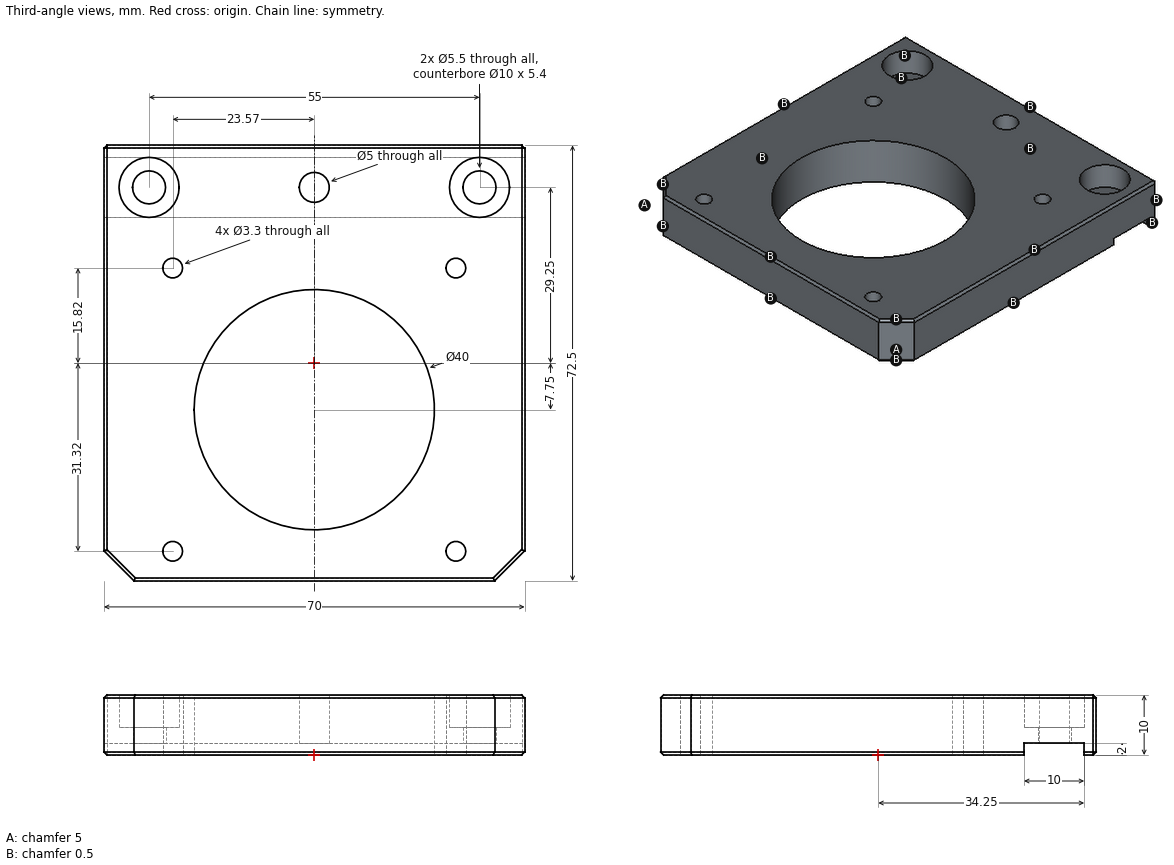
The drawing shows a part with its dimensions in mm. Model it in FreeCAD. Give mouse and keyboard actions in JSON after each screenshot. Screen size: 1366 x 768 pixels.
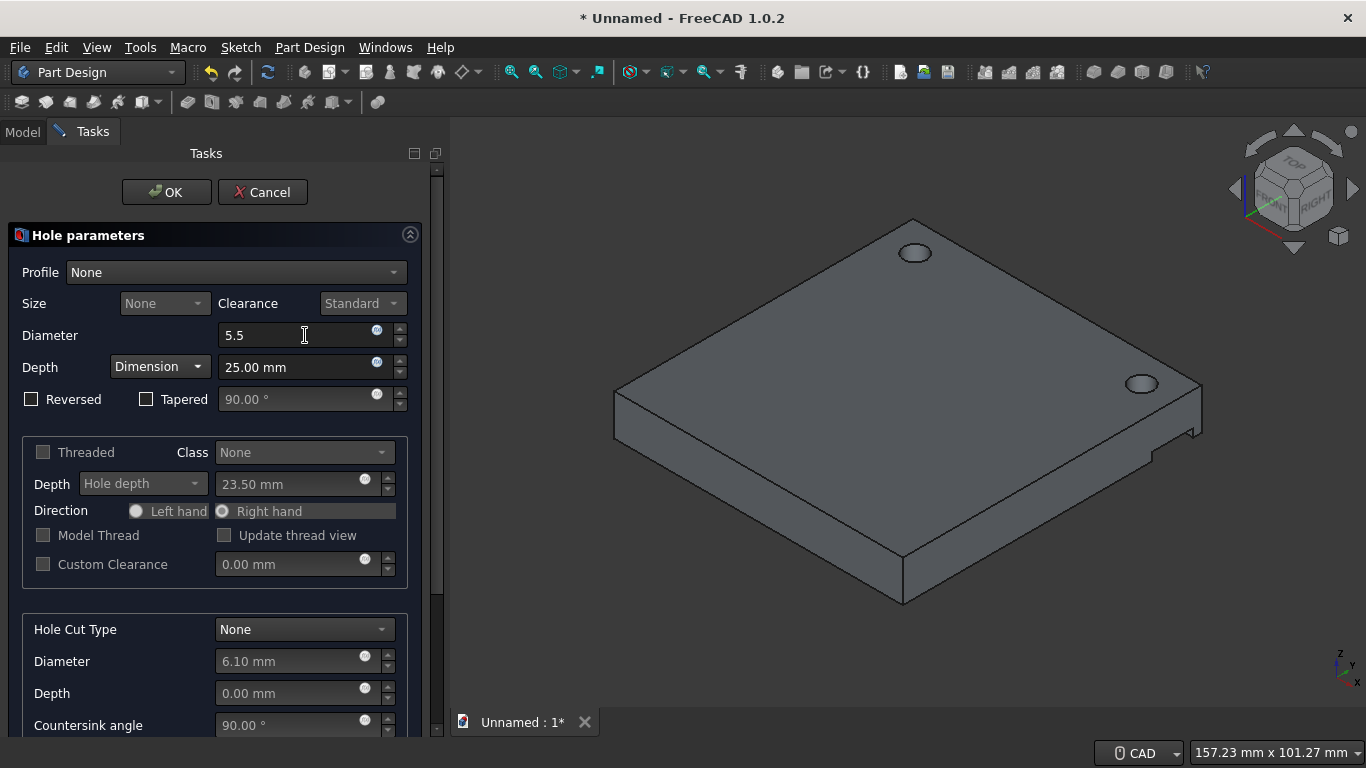
{"action": "left_click", "coordinate": [161, 366]}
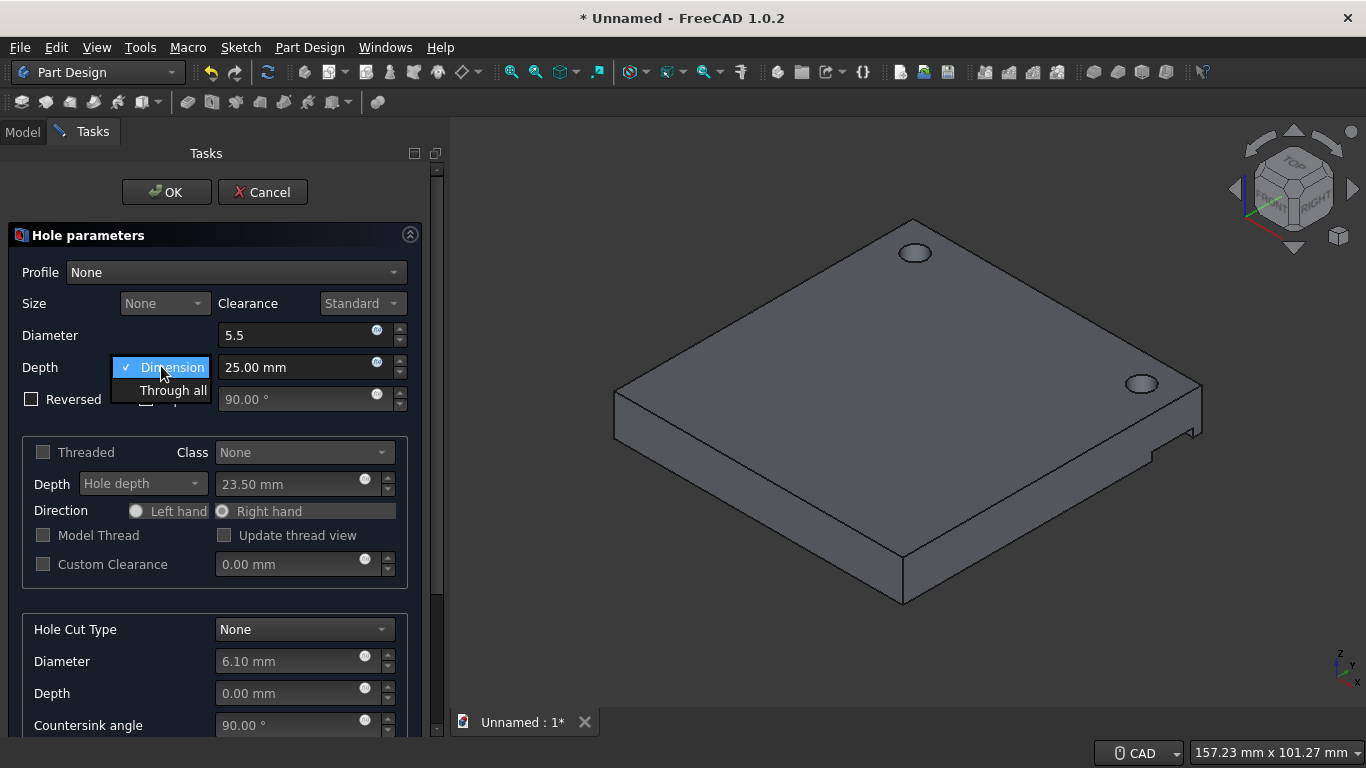
{"action": "left_click", "coordinate": [160, 390]}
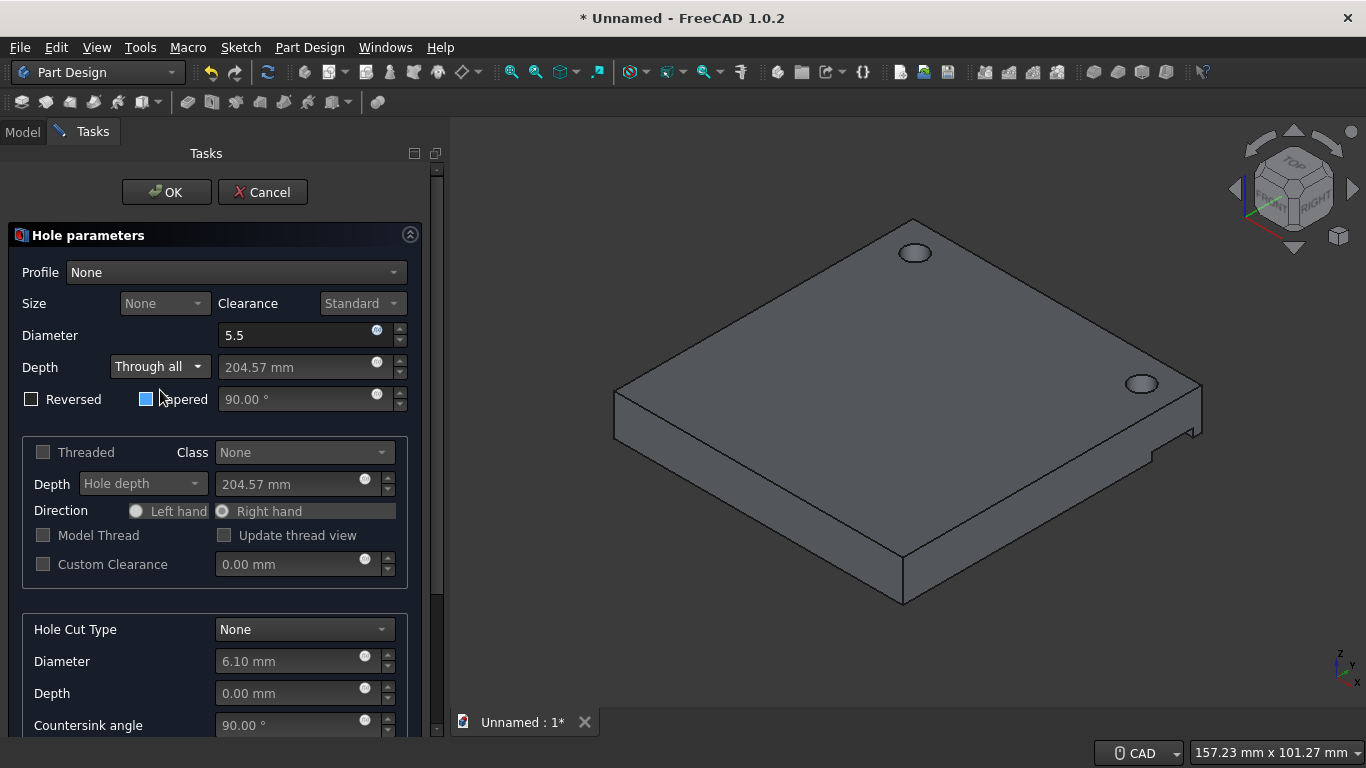
{"action": "left_click", "coordinate": [306, 630]}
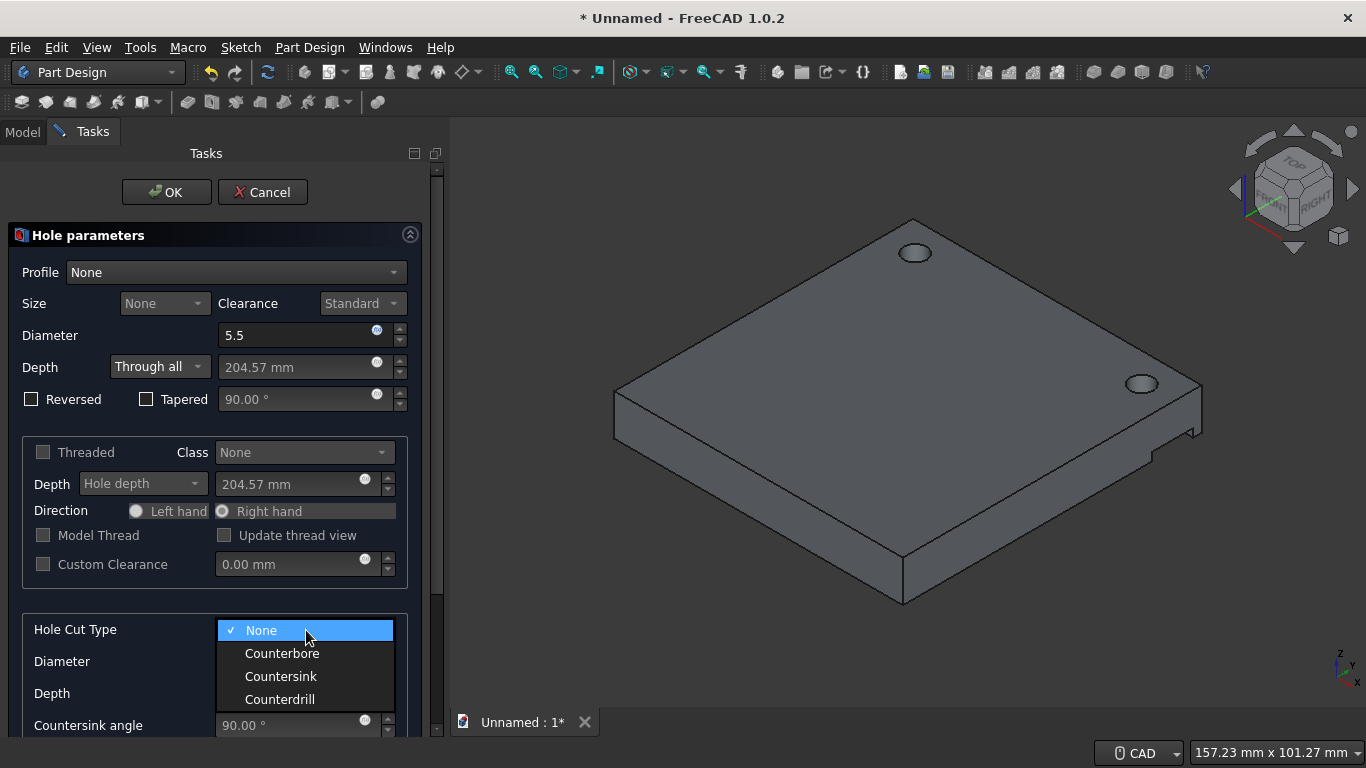
{"action": "left_click", "coordinate": [304, 654]}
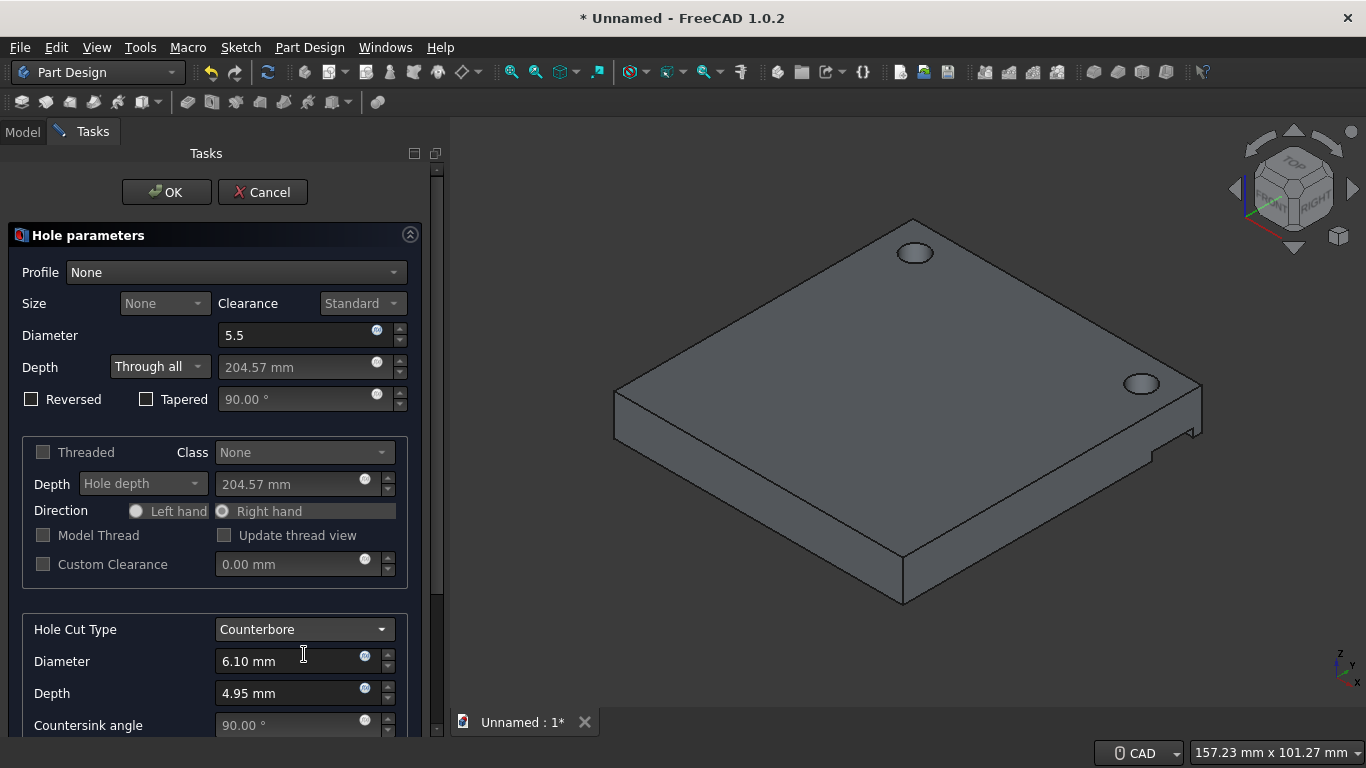
{"action": "triple_click", "coordinate": [298, 661]}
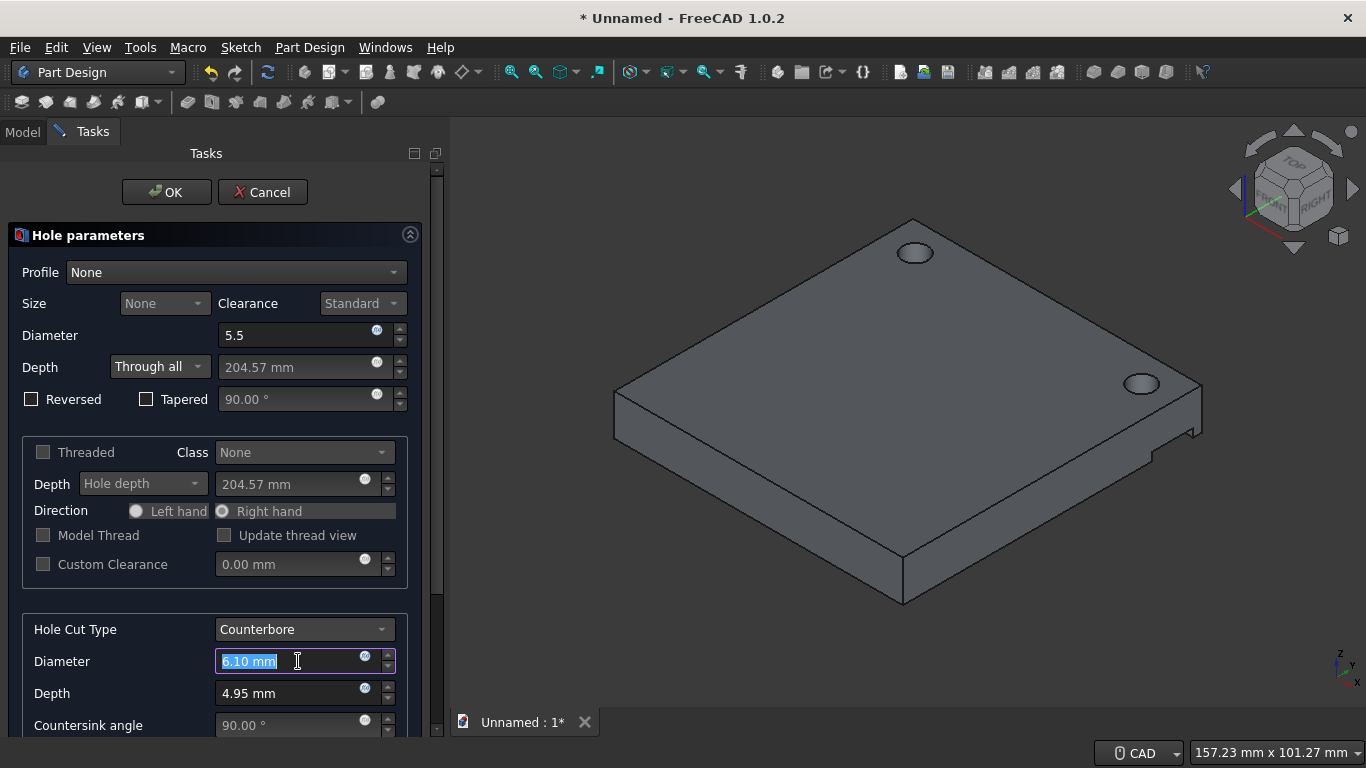
{"action": "type", "text": "10"}
{"action": "key", "text": "Tab"}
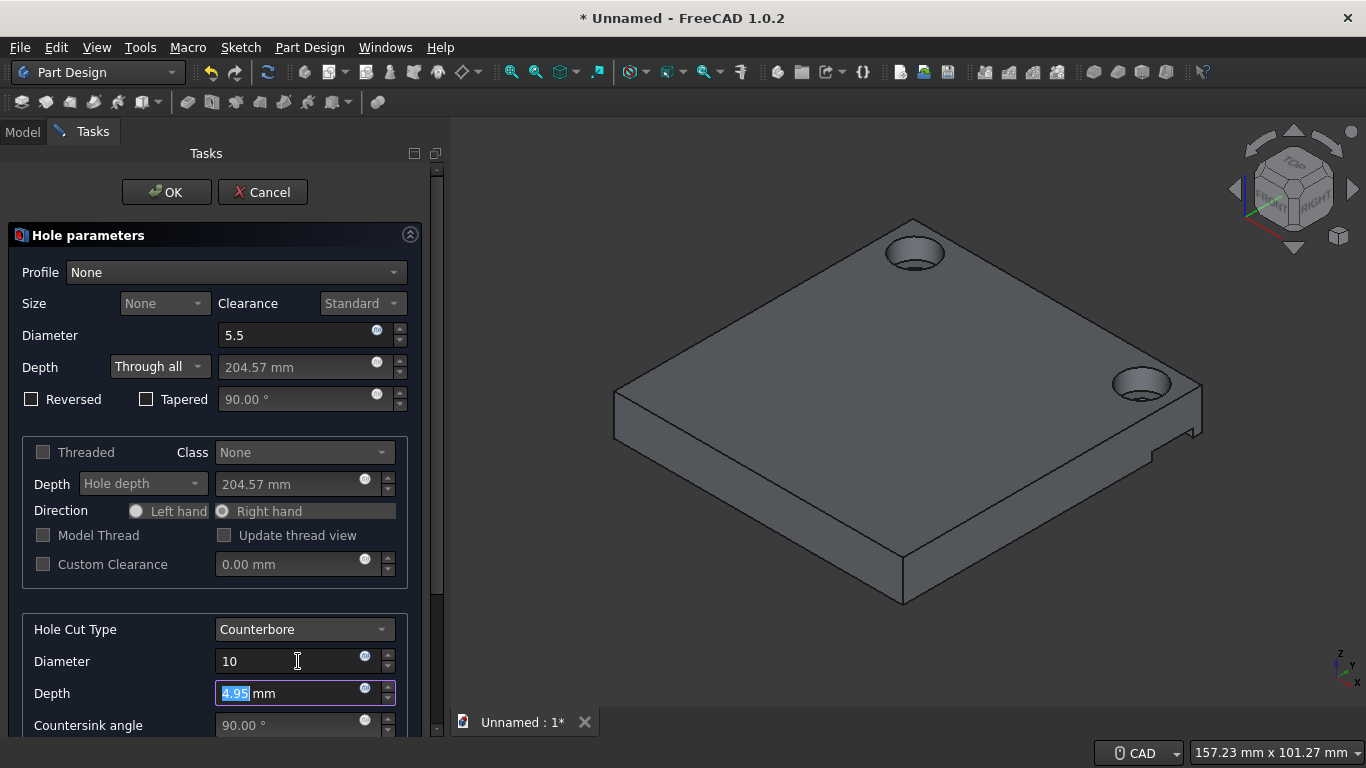
{"action": "type", "text": "5.4"}
{"action": "key", "text": "Tab"}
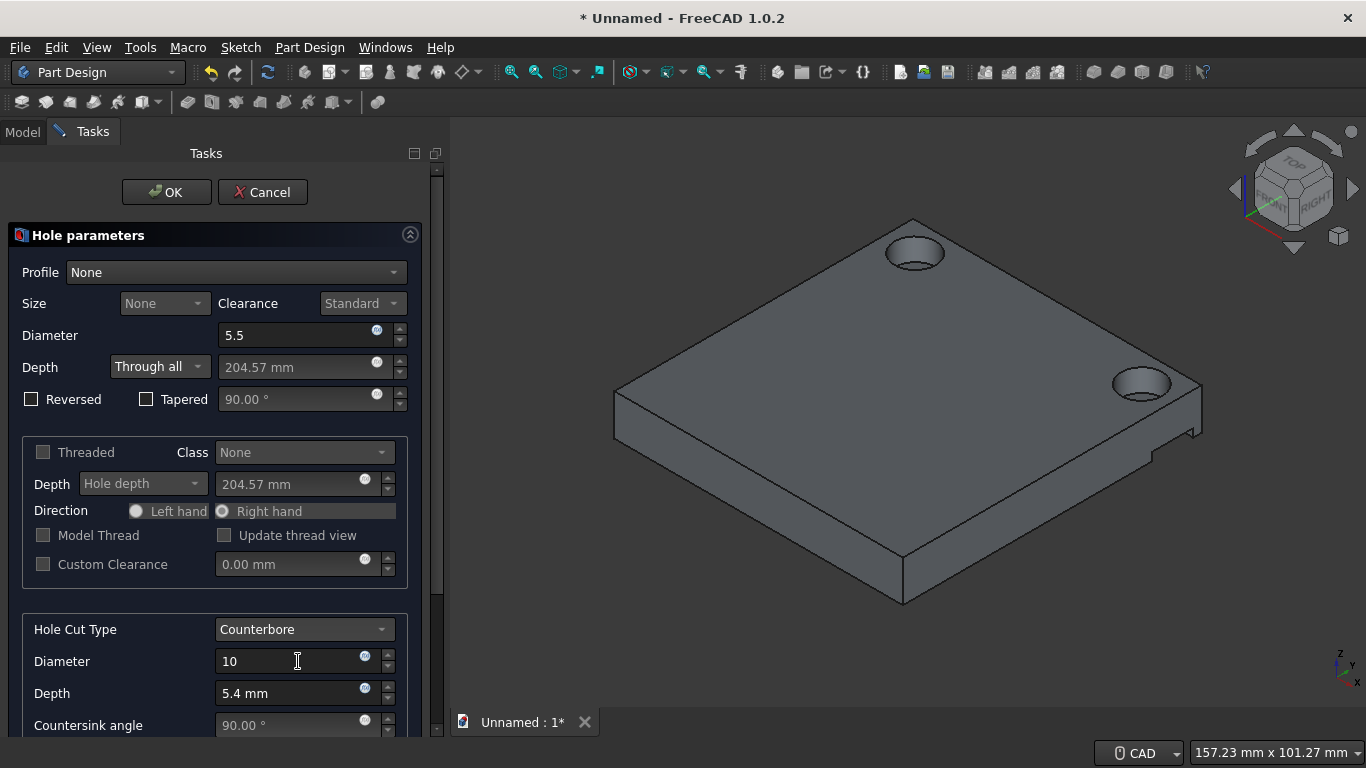
{"action": "left_click", "coordinate": [167, 192]}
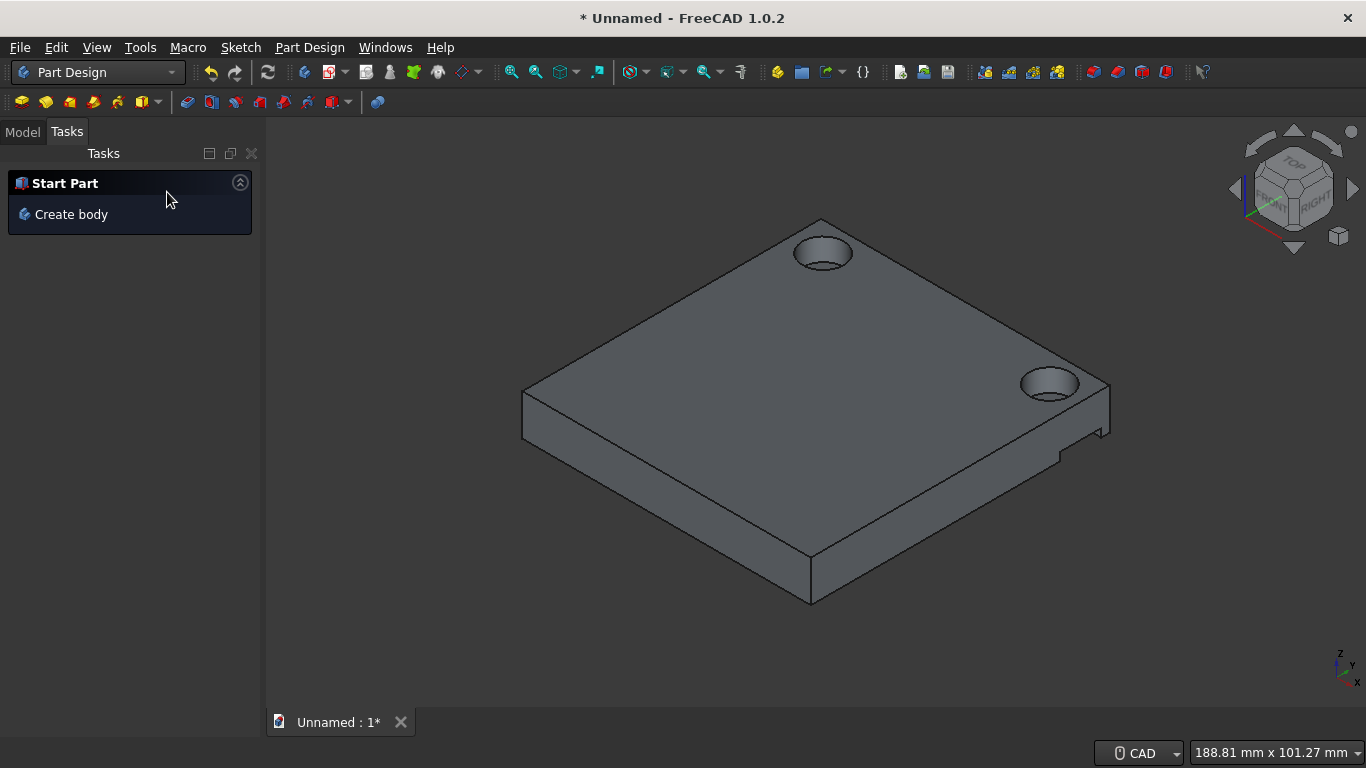
{"action": "left_click", "coordinate": [816, 387]}